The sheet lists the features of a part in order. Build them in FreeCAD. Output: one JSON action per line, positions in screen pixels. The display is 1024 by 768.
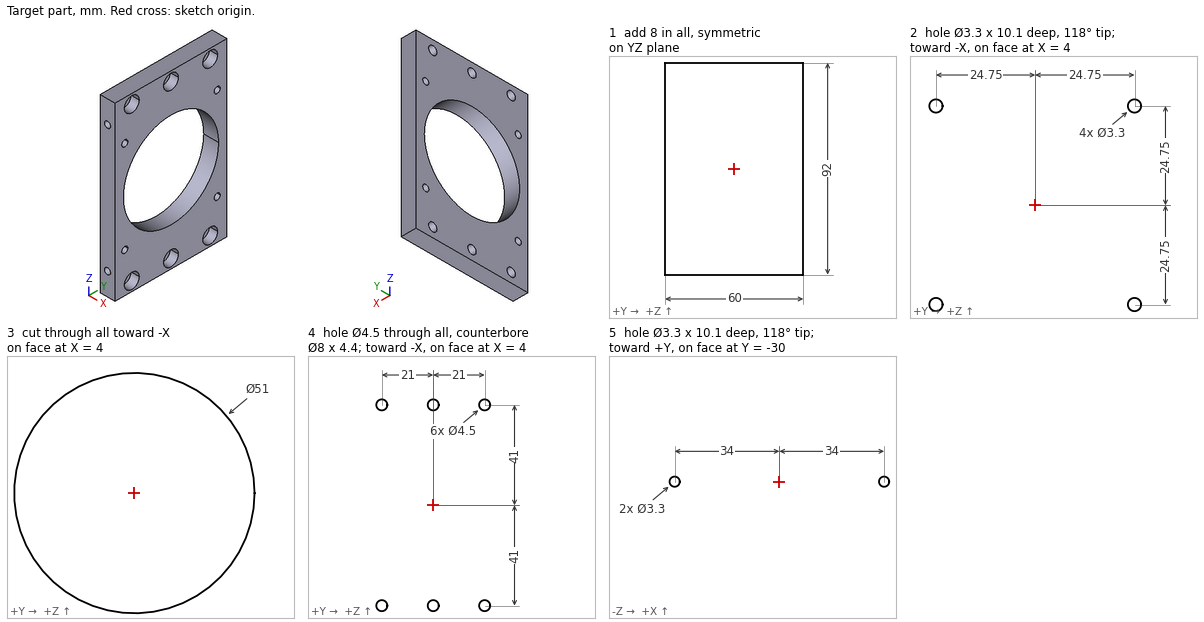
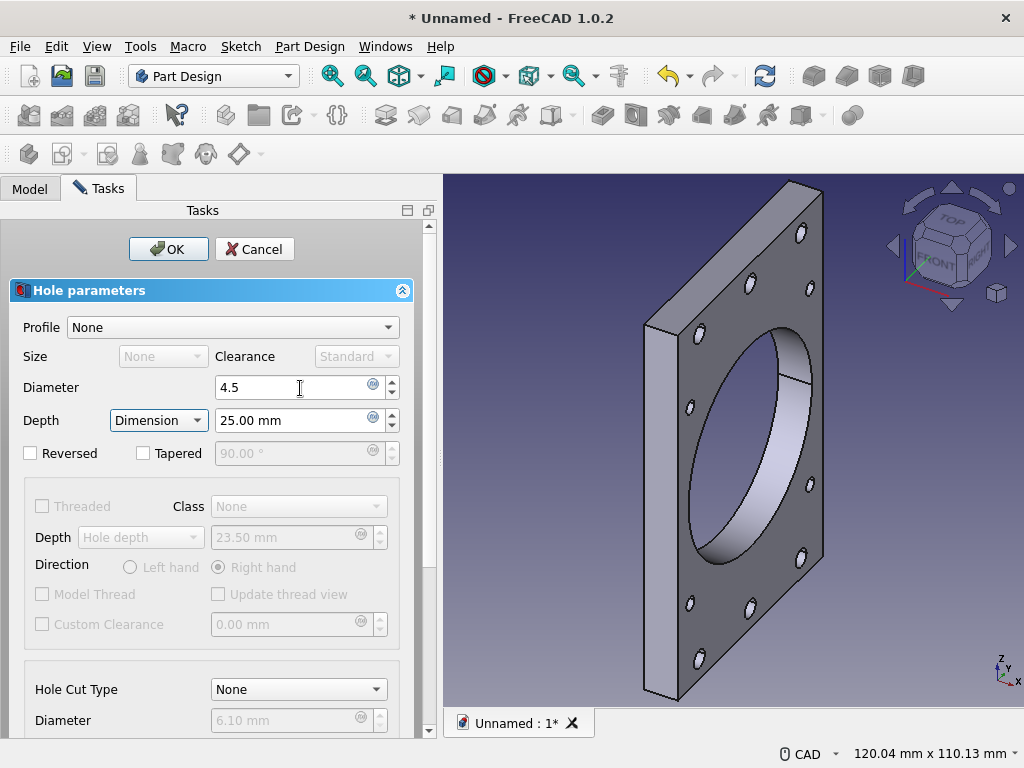
{"action": "left_click", "coordinate": [160, 420]}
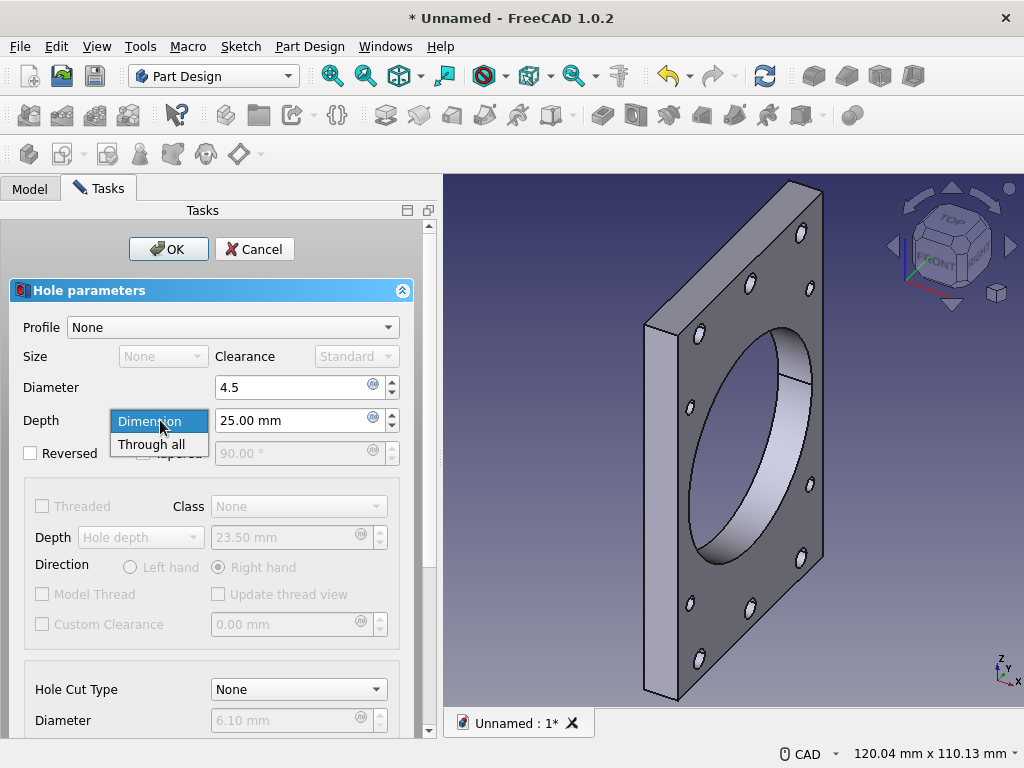
{"action": "left_click", "coordinate": [158, 444]}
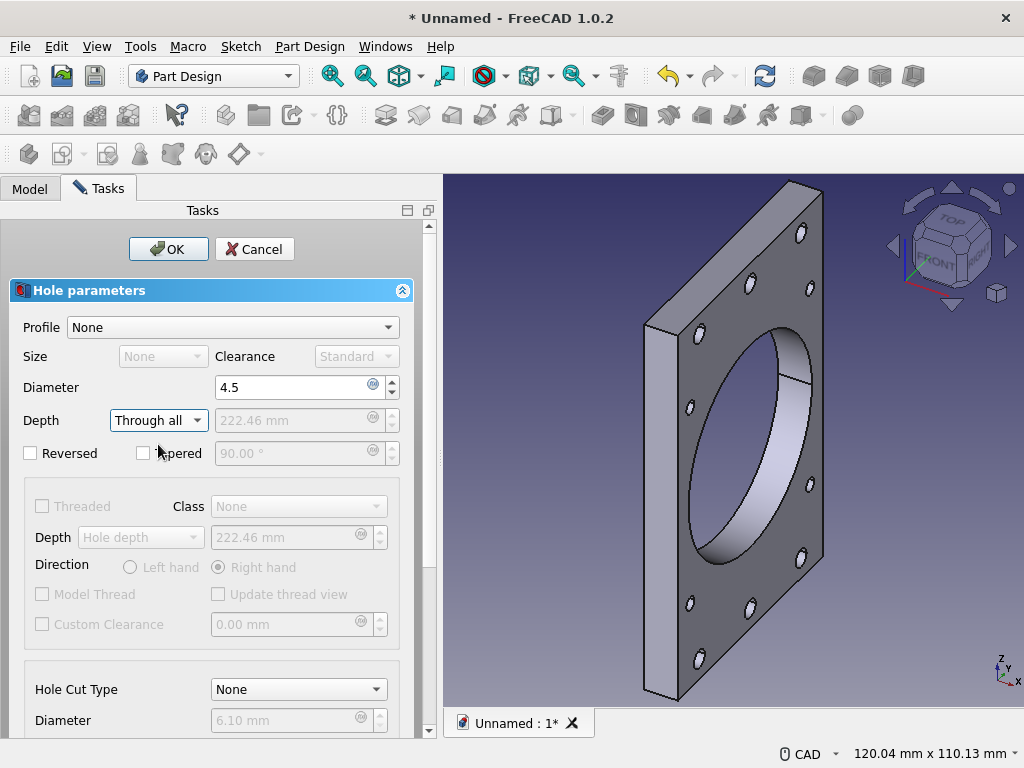
{"action": "left_click", "coordinate": [300, 690]}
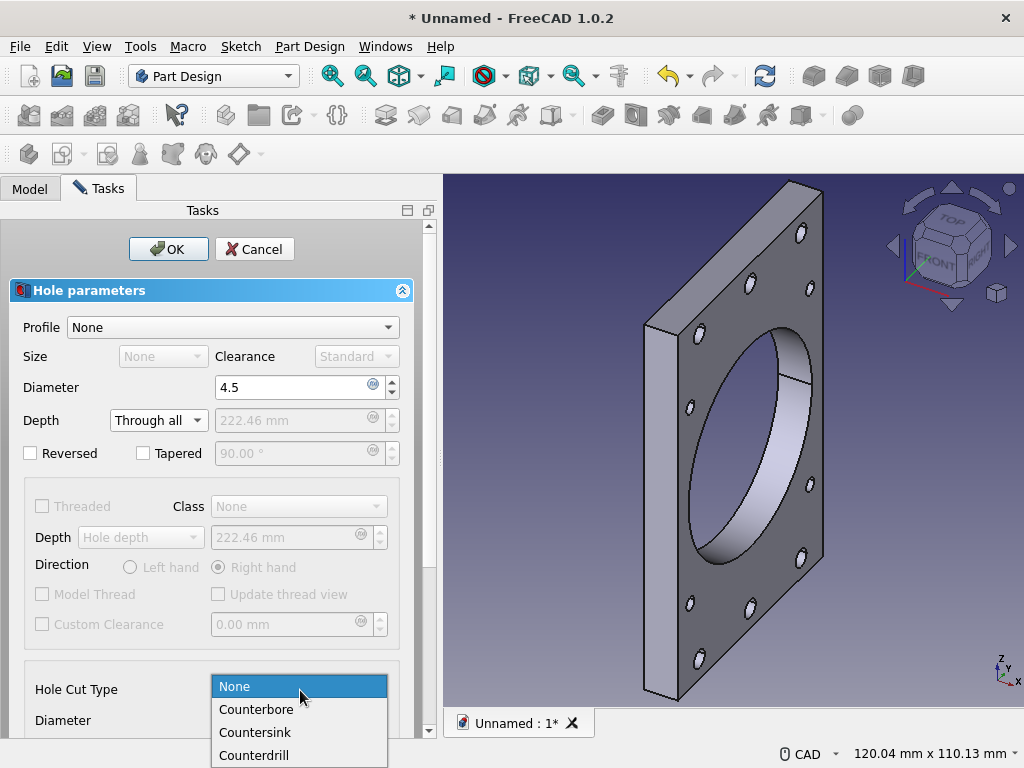
{"action": "left_click", "coordinate": [298, 710]}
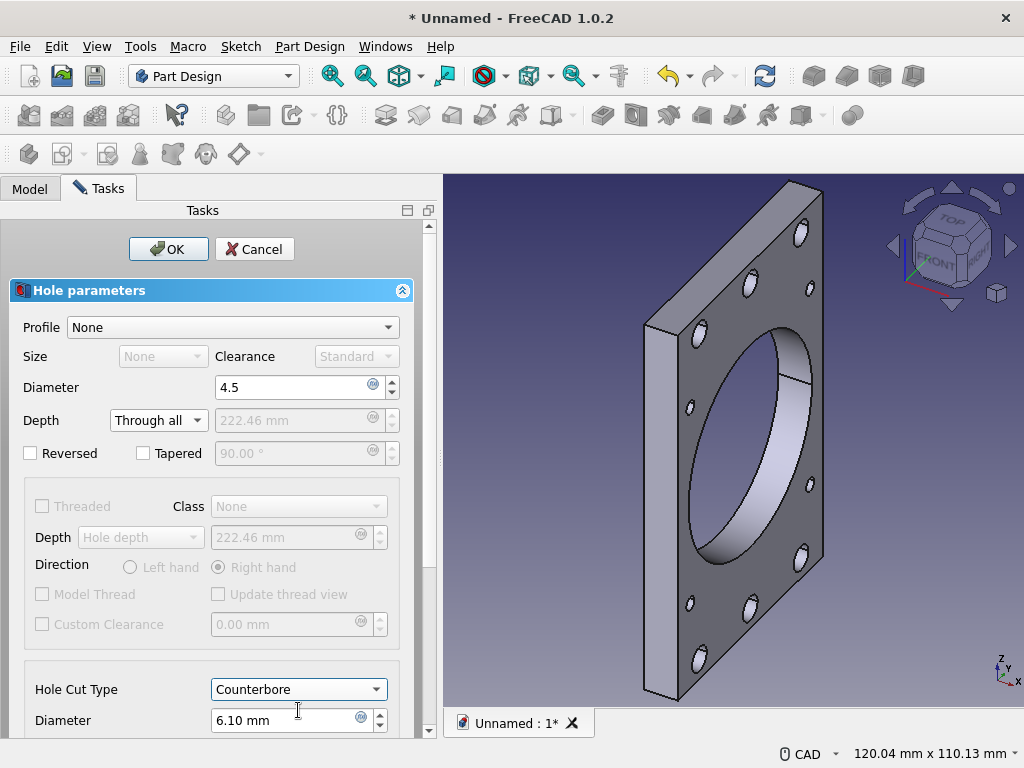
{"action": "triple_click", "coordinate": [292, 720]}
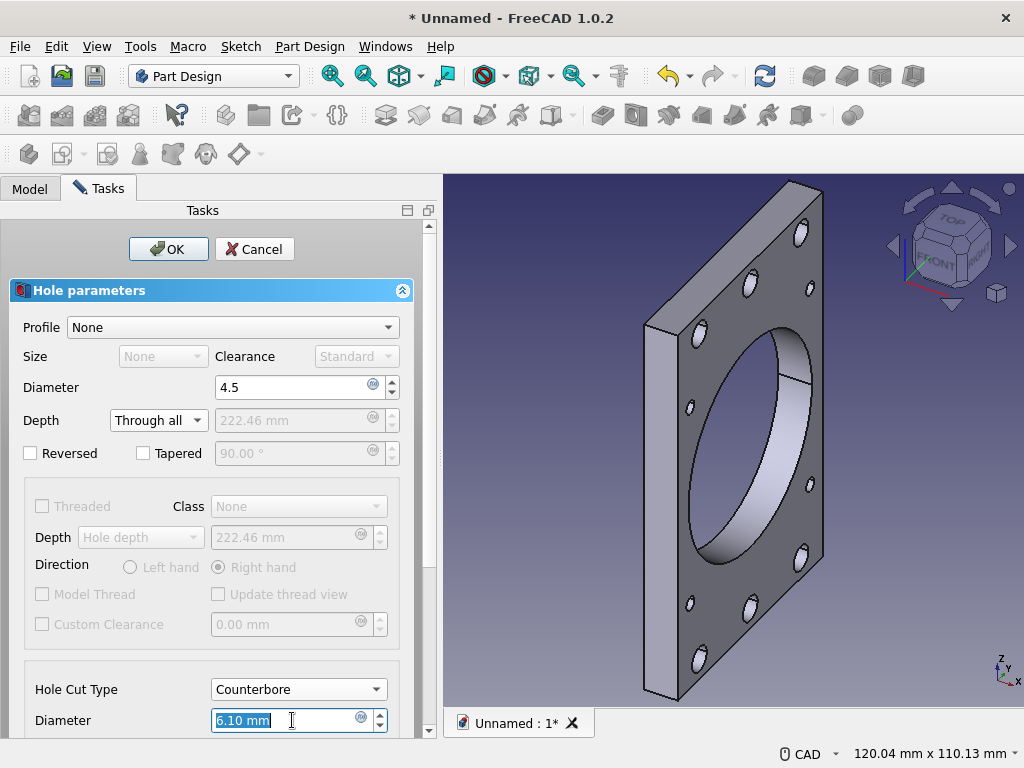
{"action": "type", "text": "8"}
{"action": "key", "text": "Tab"}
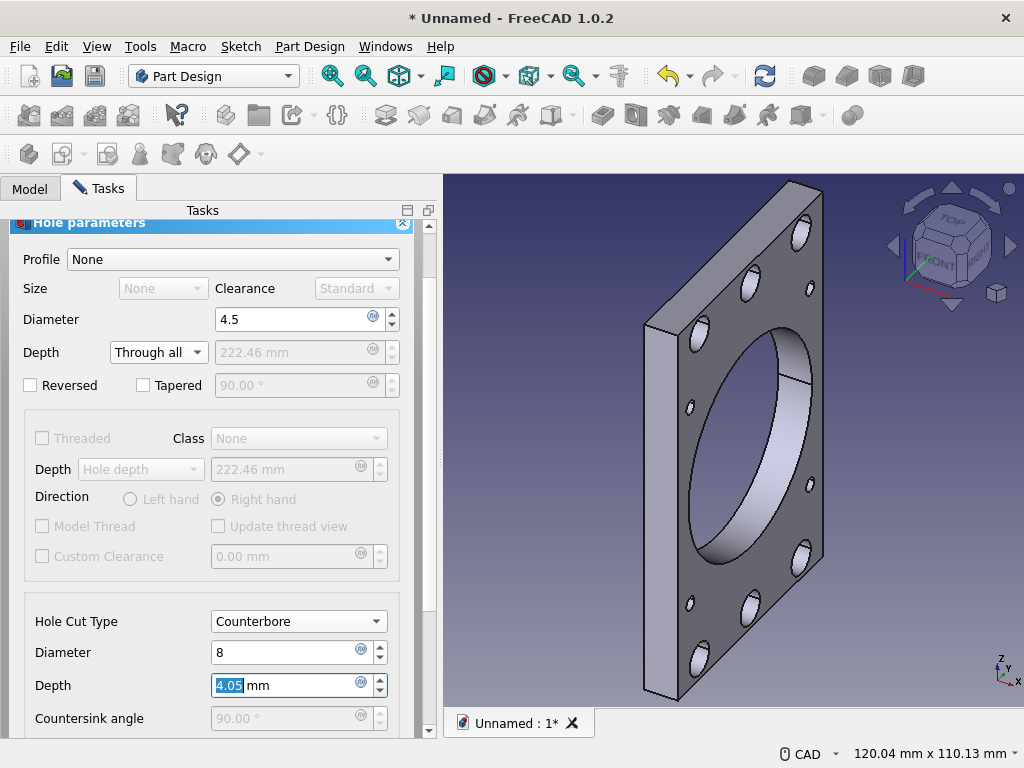
{"action": "type", "text": "4.4"}
{"action": "key", "text": "Tab"}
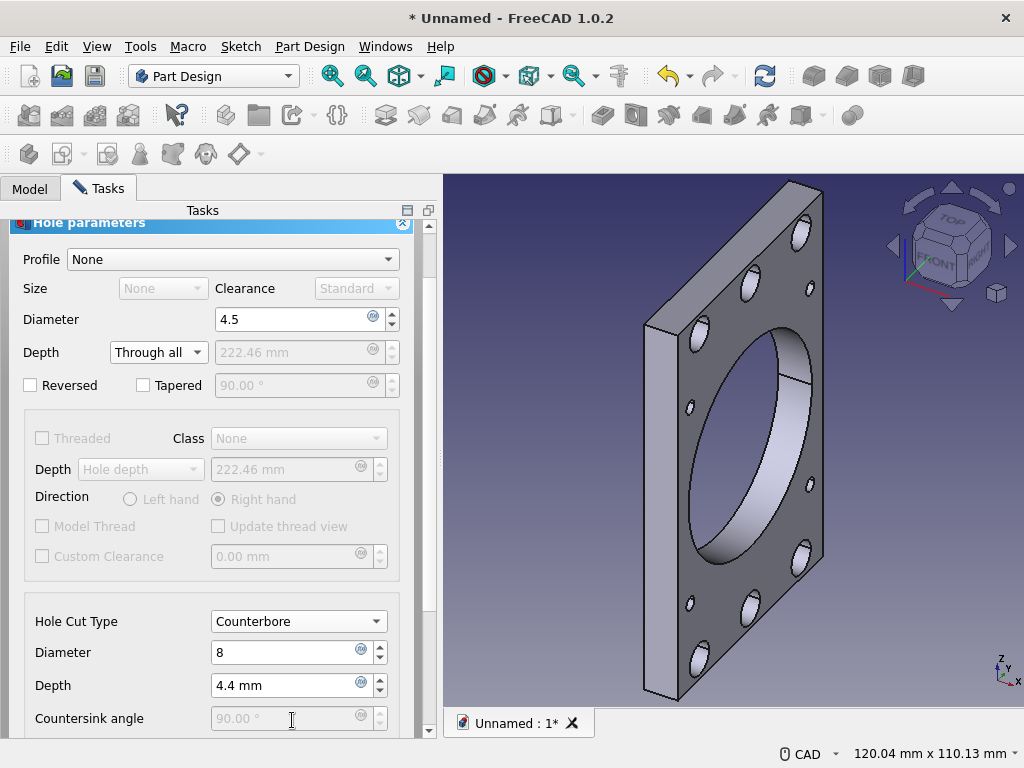
{"action": "scroll", "coordinate": [429, 479], "scroll_direction": "up", "scroll_amount": 2}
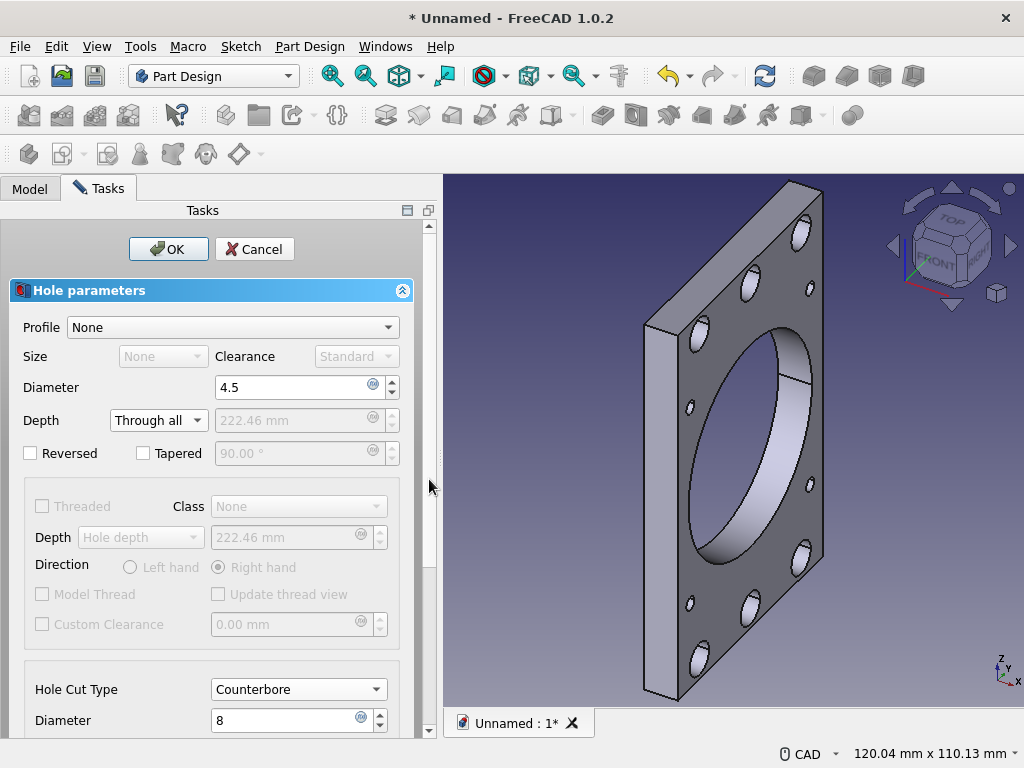
{"action": "left_click", "coordinate": [169, 249]}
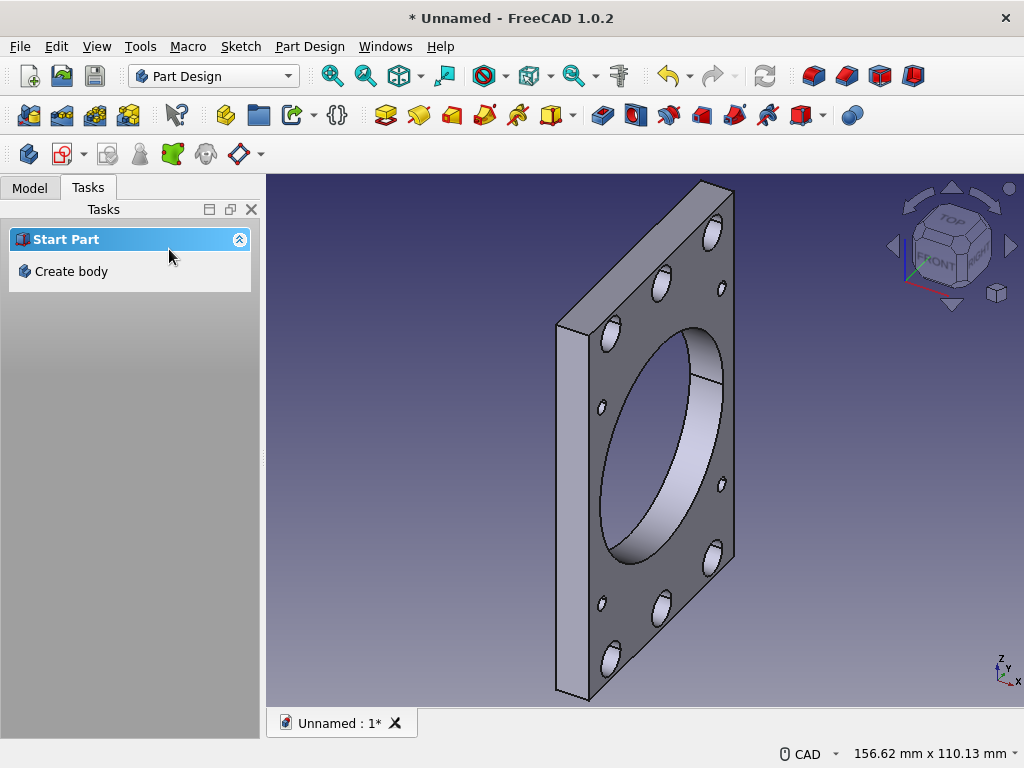
{"action": "left_click", "coordinate": [572, 564]}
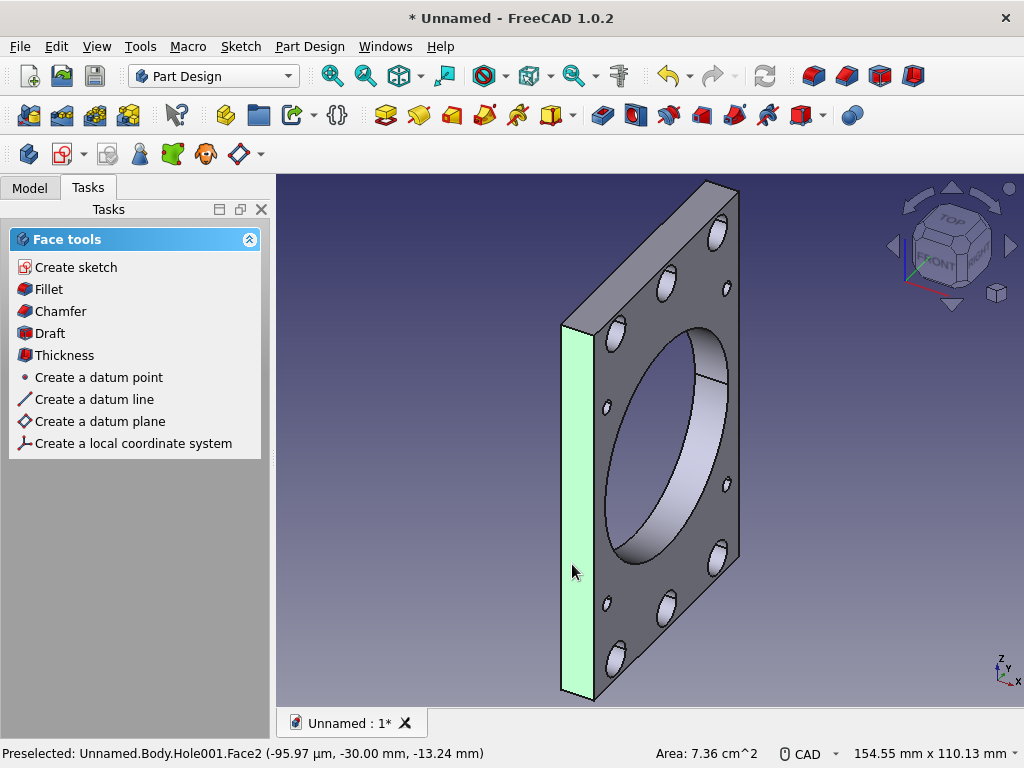
{"action": "left_click", "coordinate": [62, 154]}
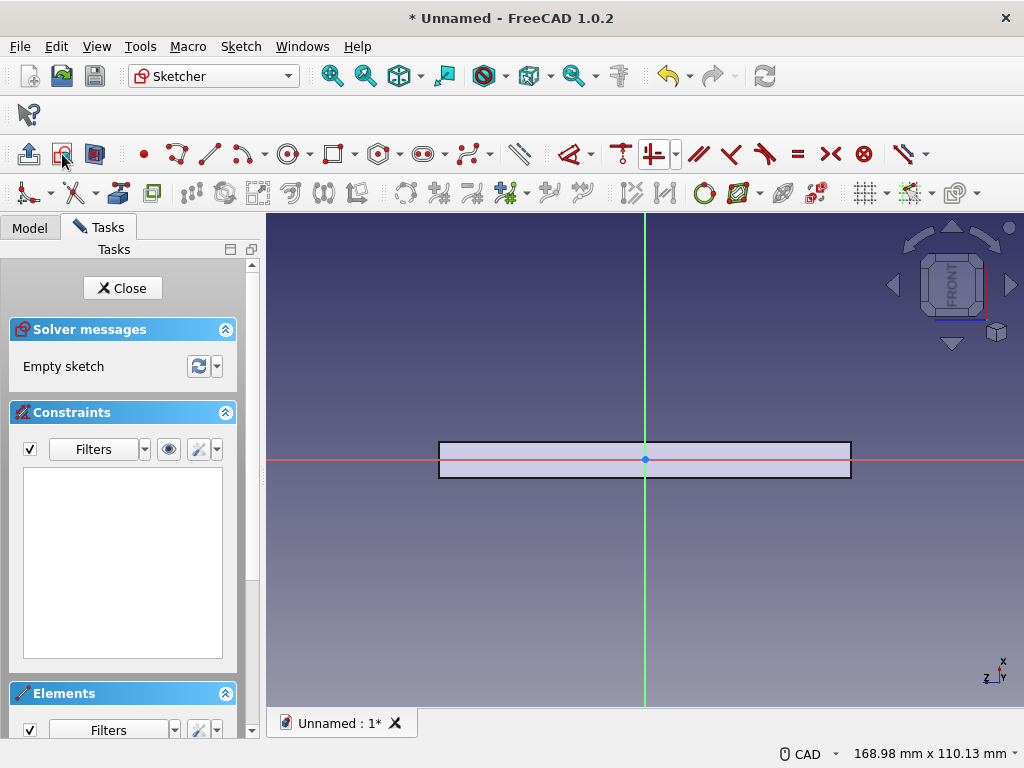
{"action": "left_click", "coordinate": [288, 154]}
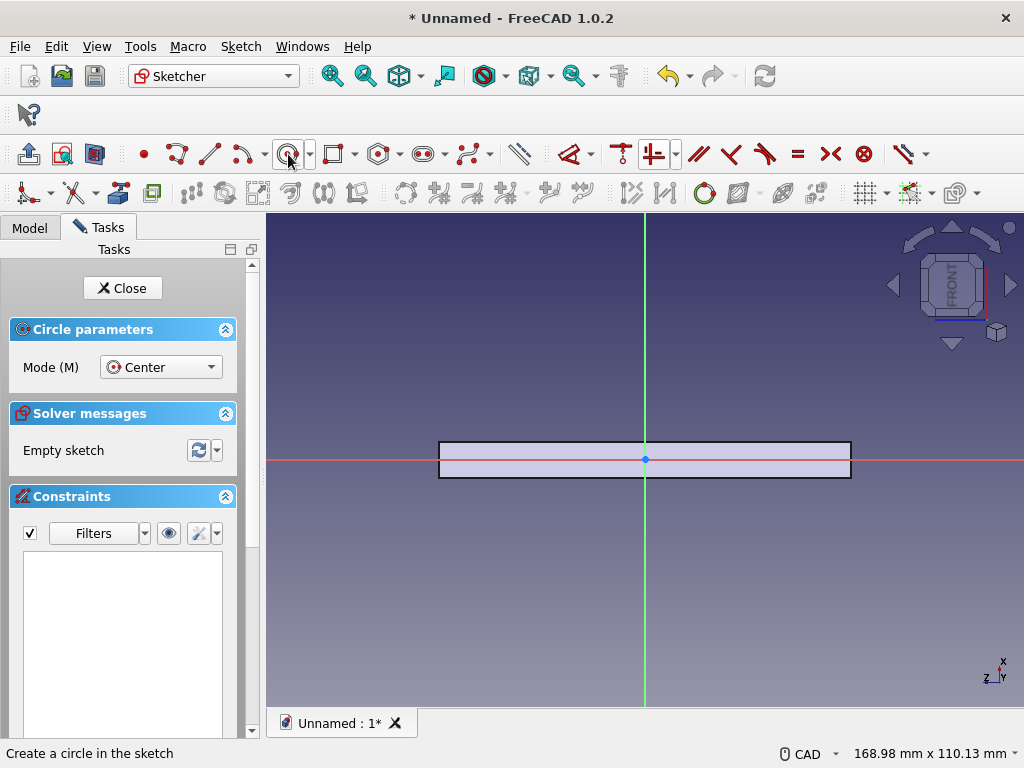
{"action": "scroll", "coordinate": [492, 460], "scroll_direction": "up", "scroll_amount": 6}